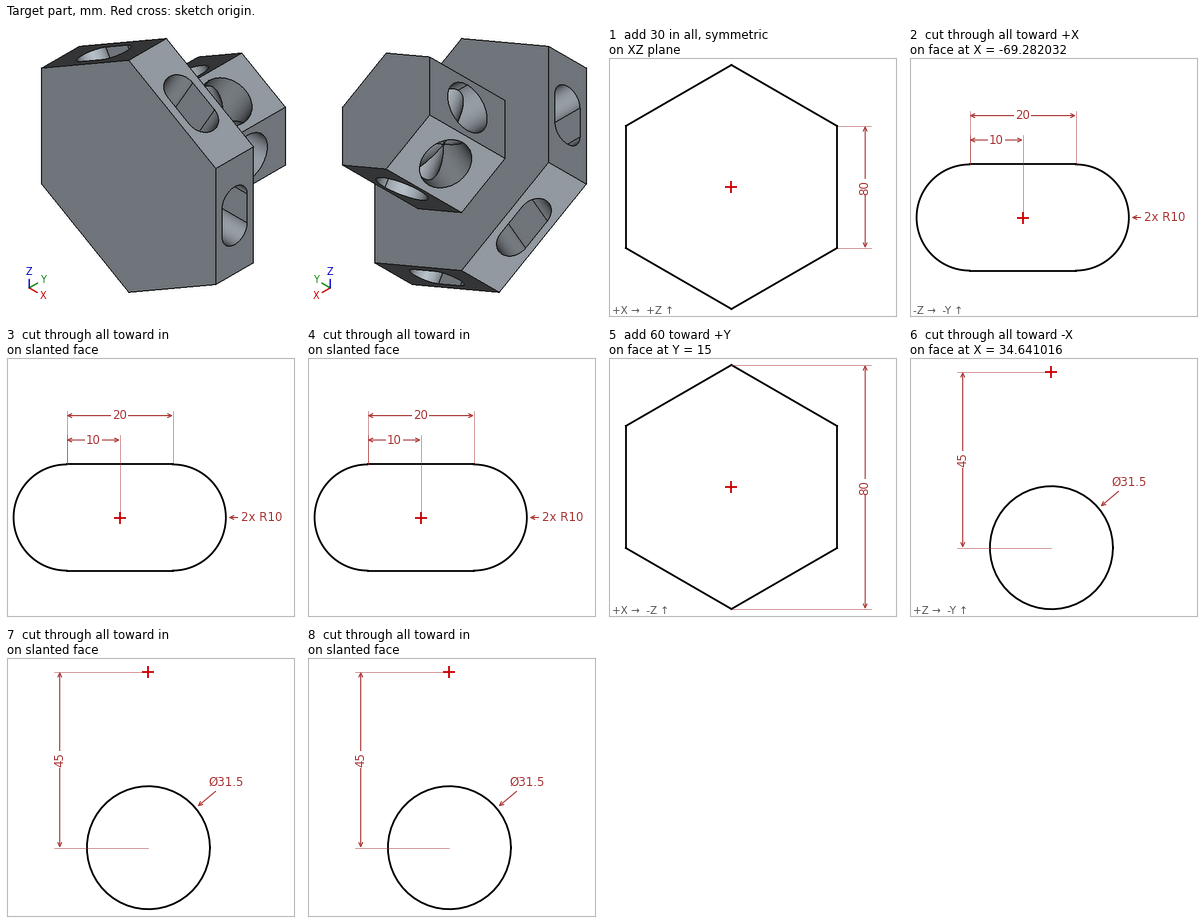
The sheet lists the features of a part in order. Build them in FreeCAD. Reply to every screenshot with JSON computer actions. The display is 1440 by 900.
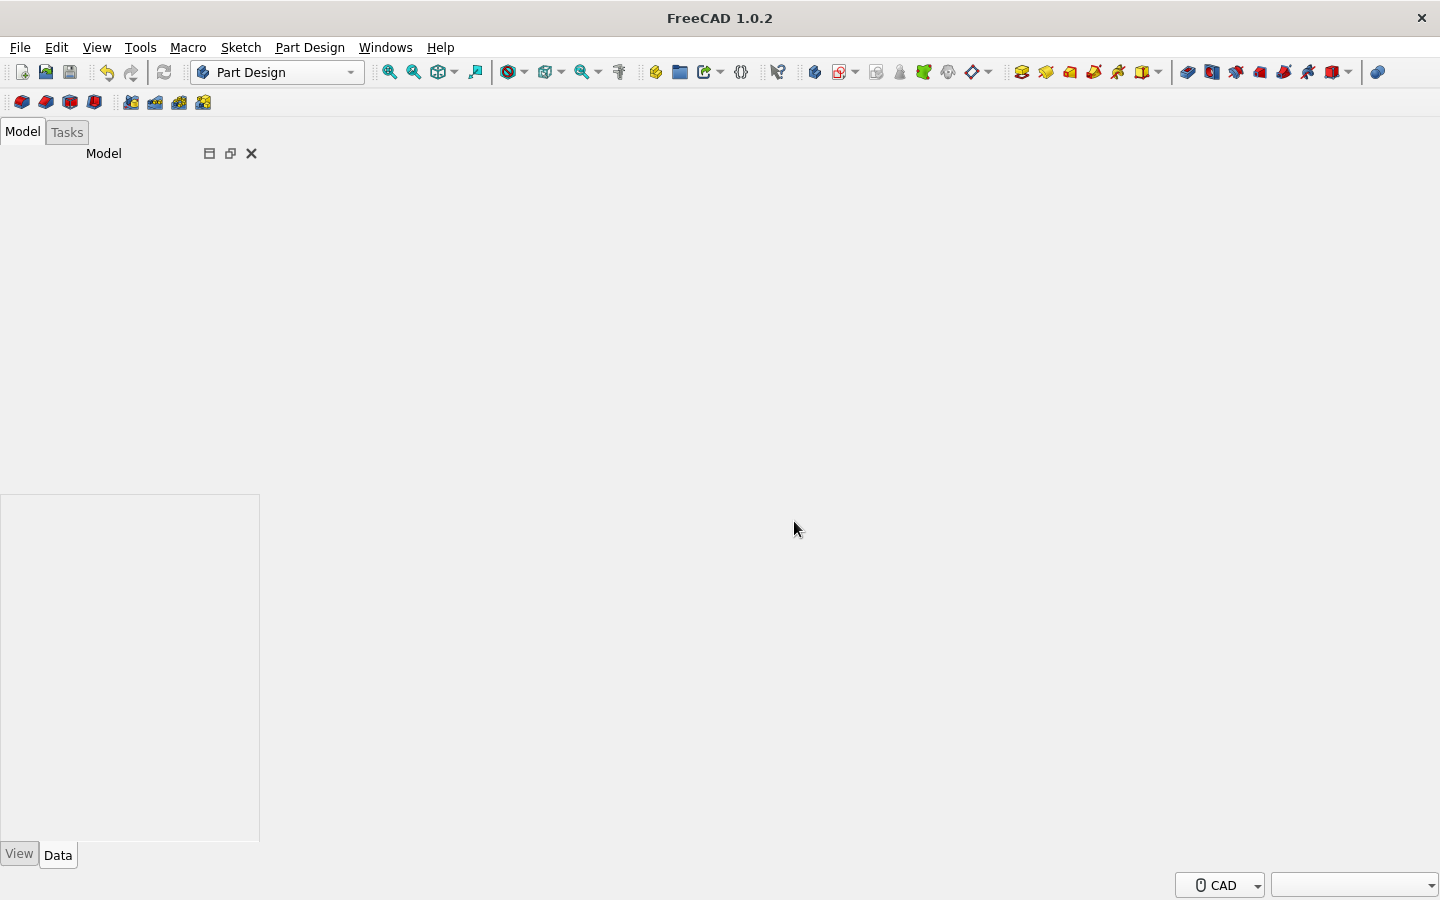
{"action": "left_click", "coordinate": [22, 72]}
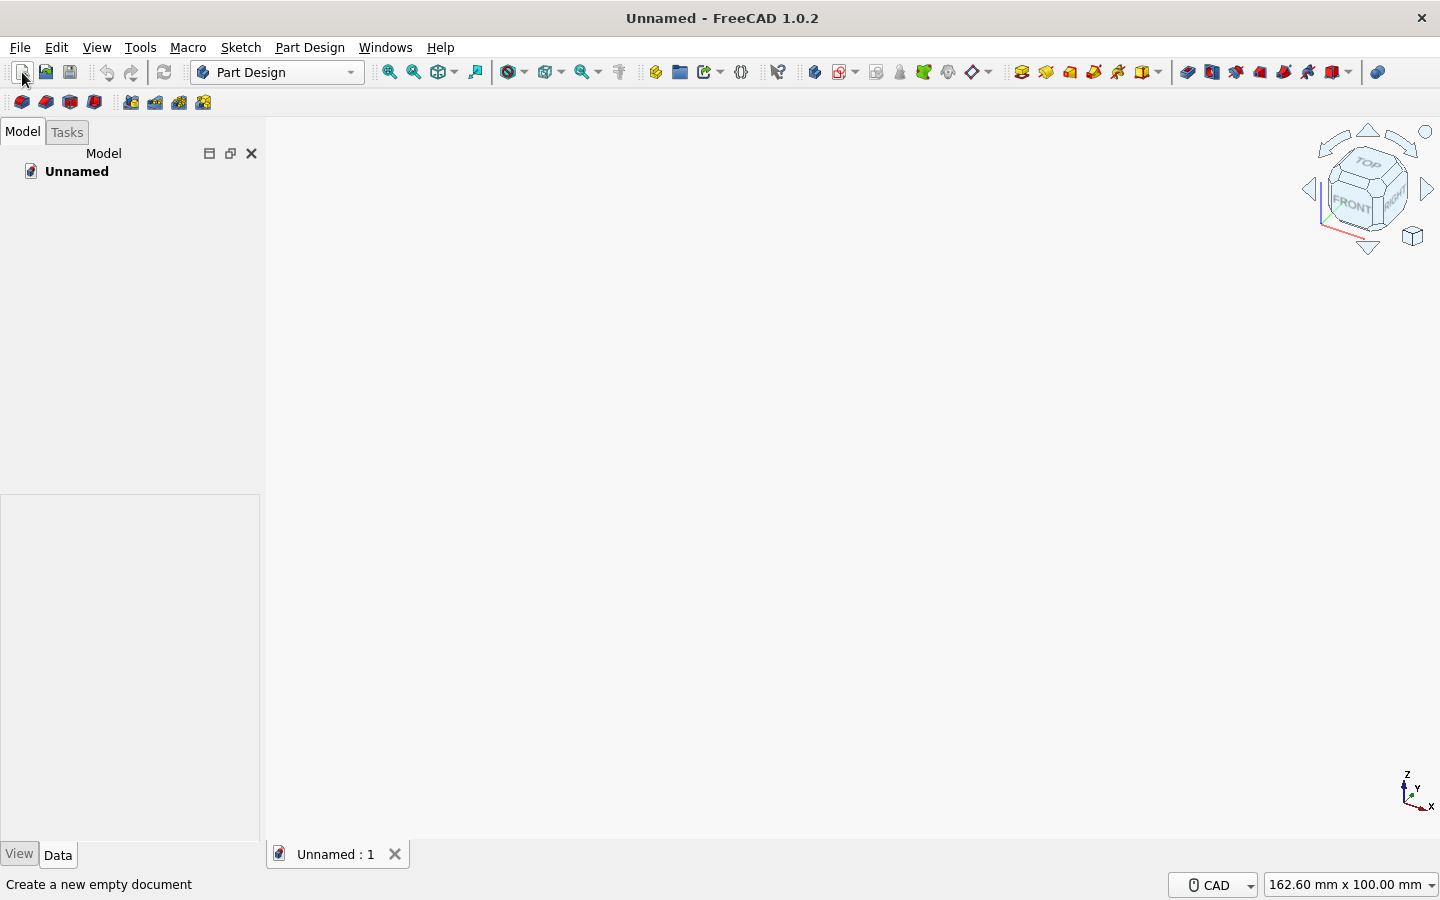
{"action": "left_click", "coordinate": [840, 72]}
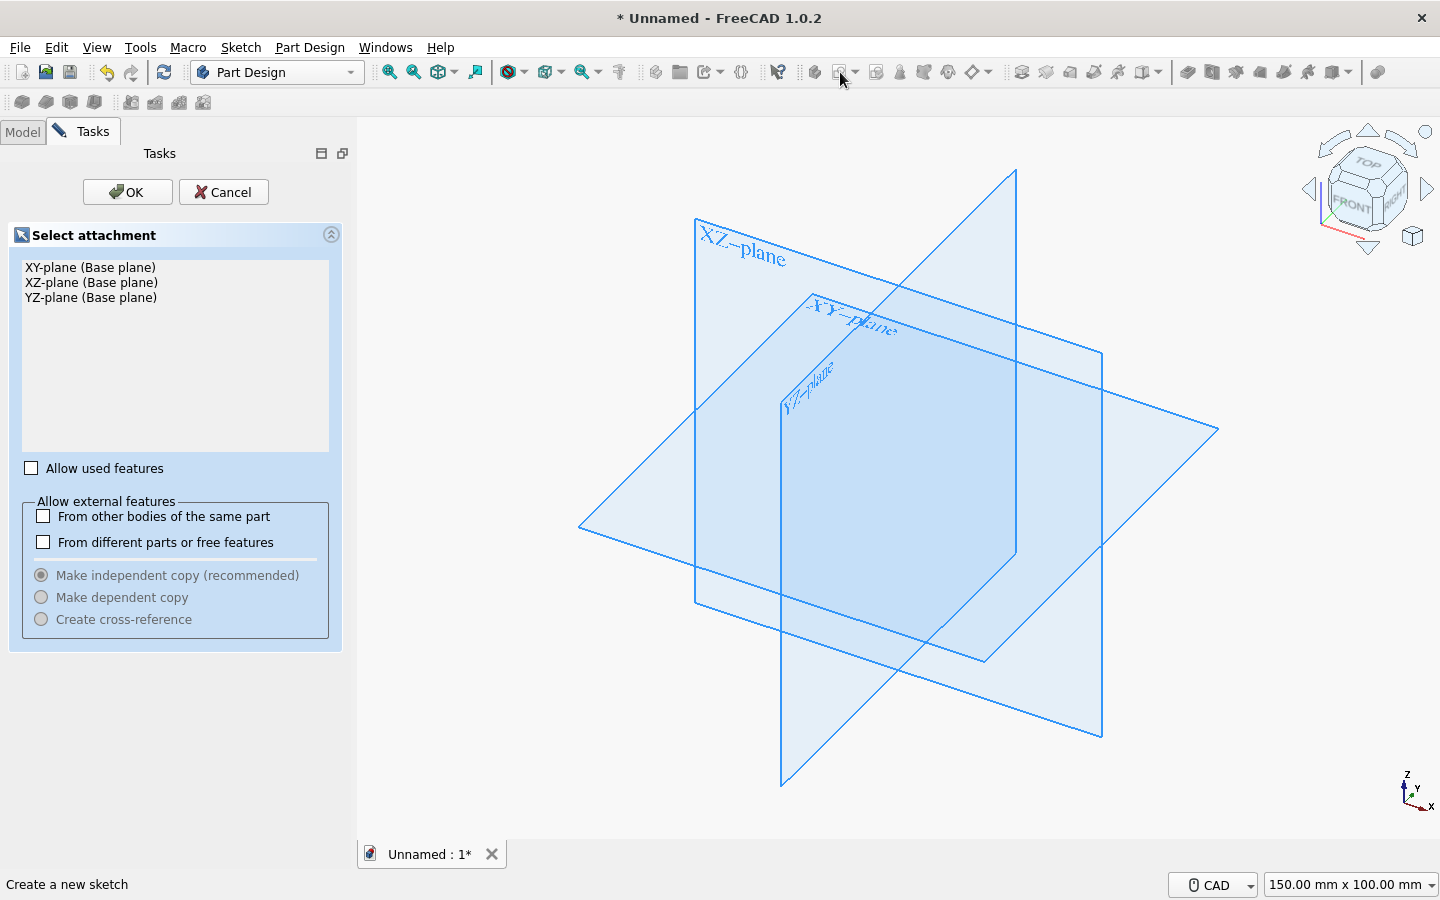
{"action": "left_click", "coordinate": [82, 282]}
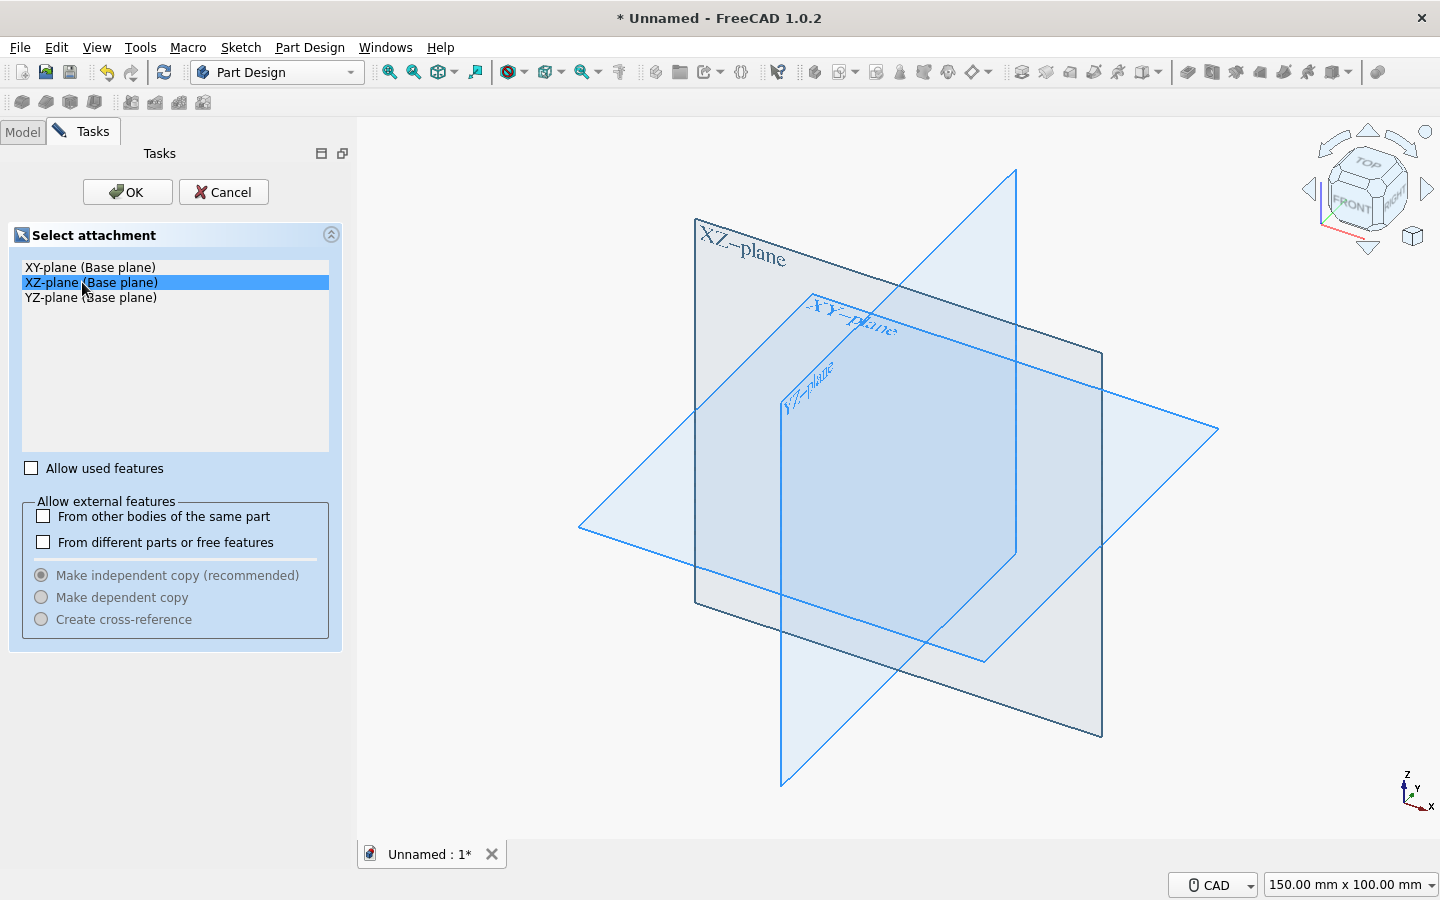
{"action": "left_click", "coordinate": [128, 192]}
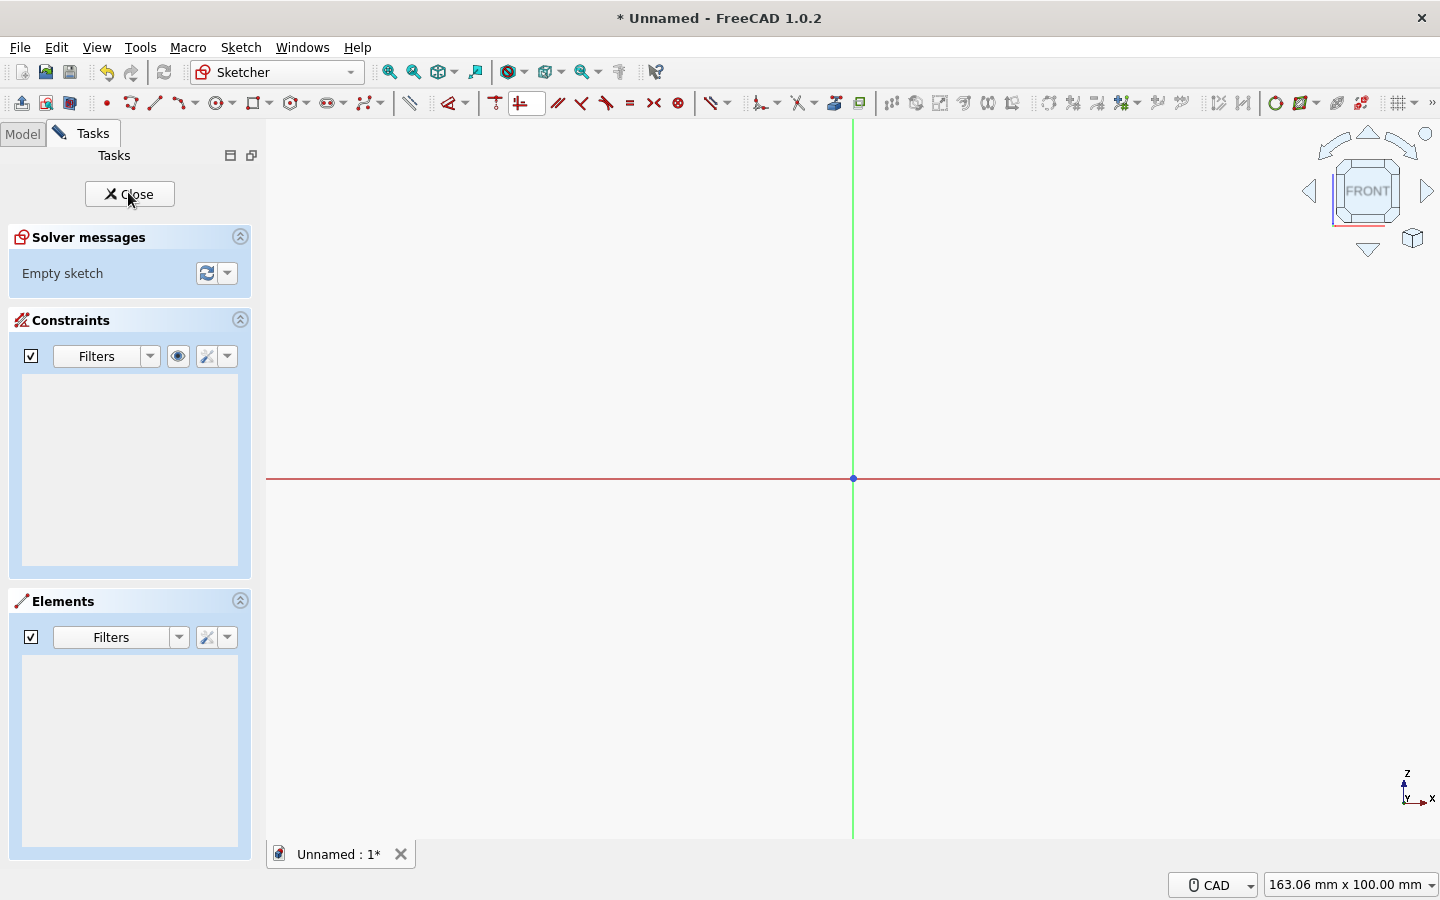
{"action": "scroll", "coordinate": [729, 479], "scroll_direction": "down", "scroll_amount": 4}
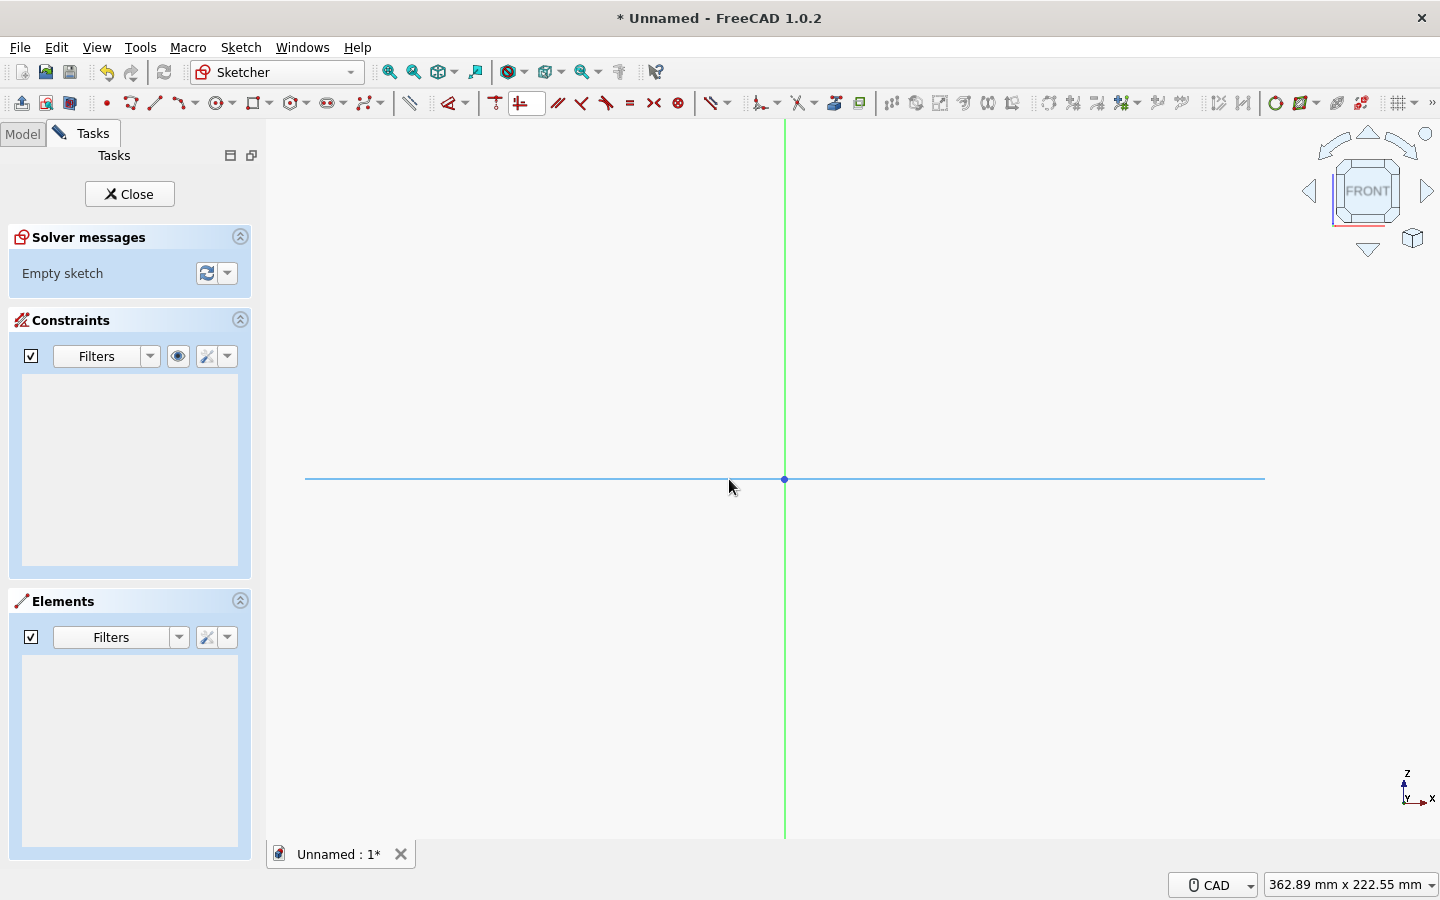
{"action": "left_click", "coordinate": [290, 104]}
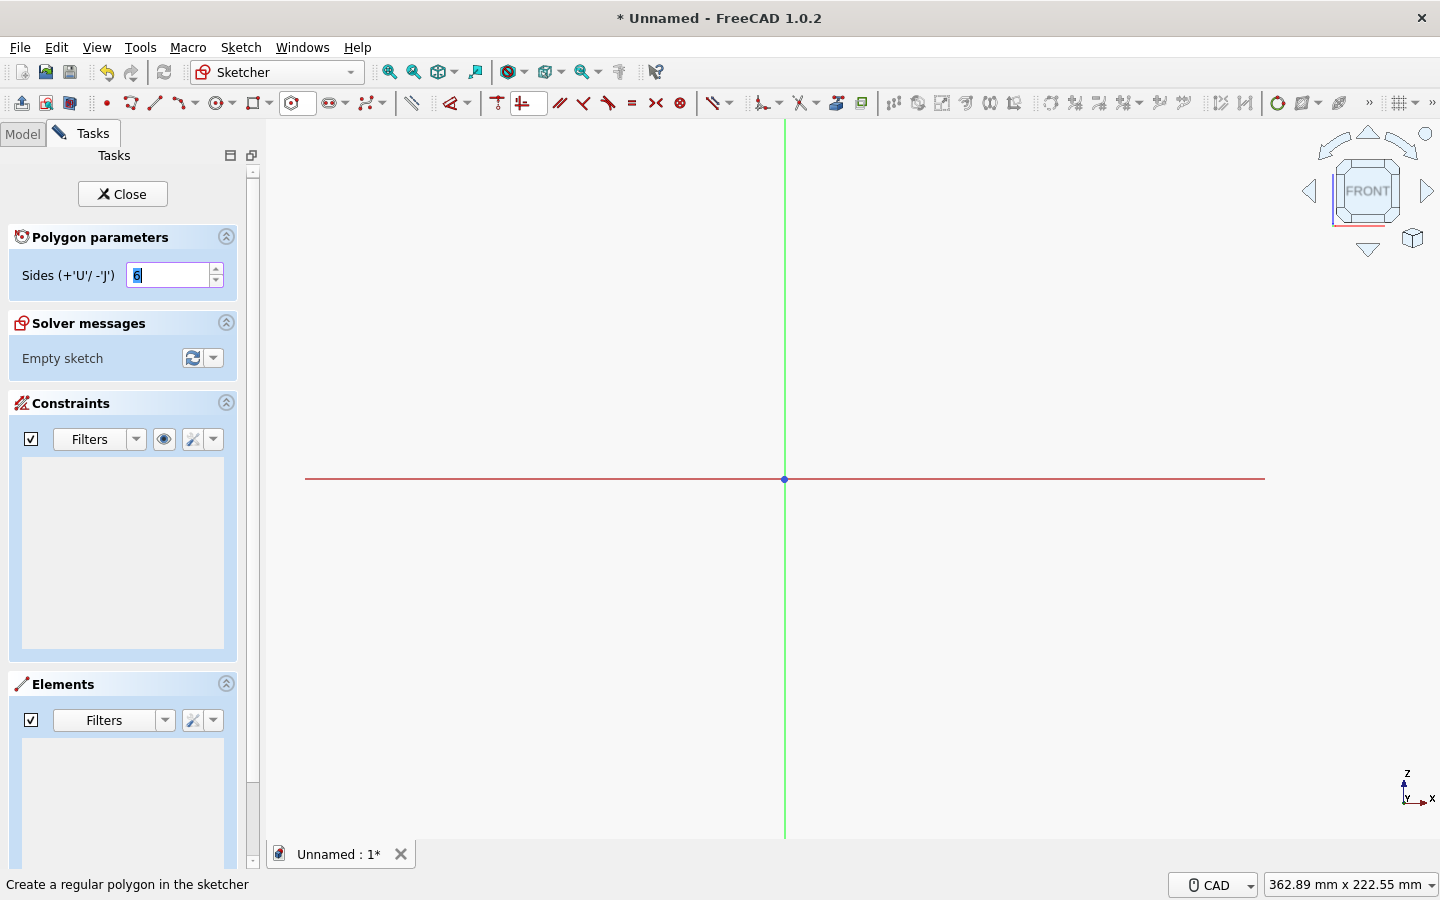
{"action": "left_click", "coordinate": [785, 479]}